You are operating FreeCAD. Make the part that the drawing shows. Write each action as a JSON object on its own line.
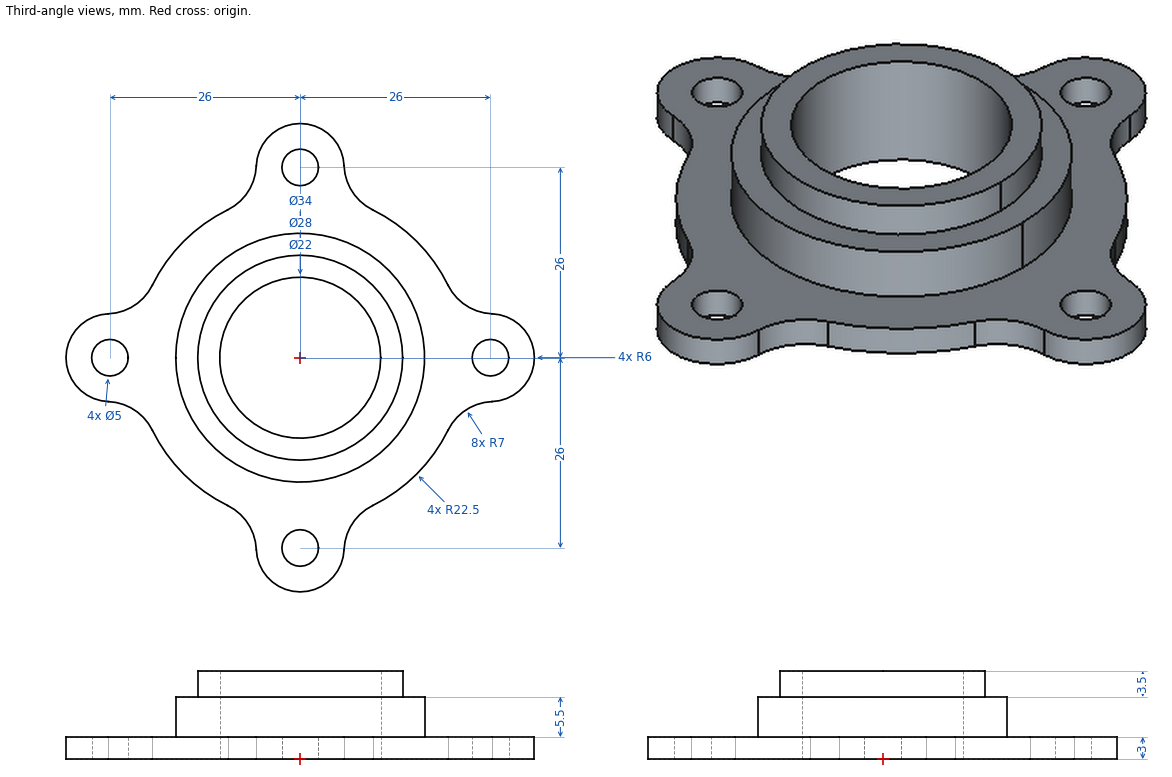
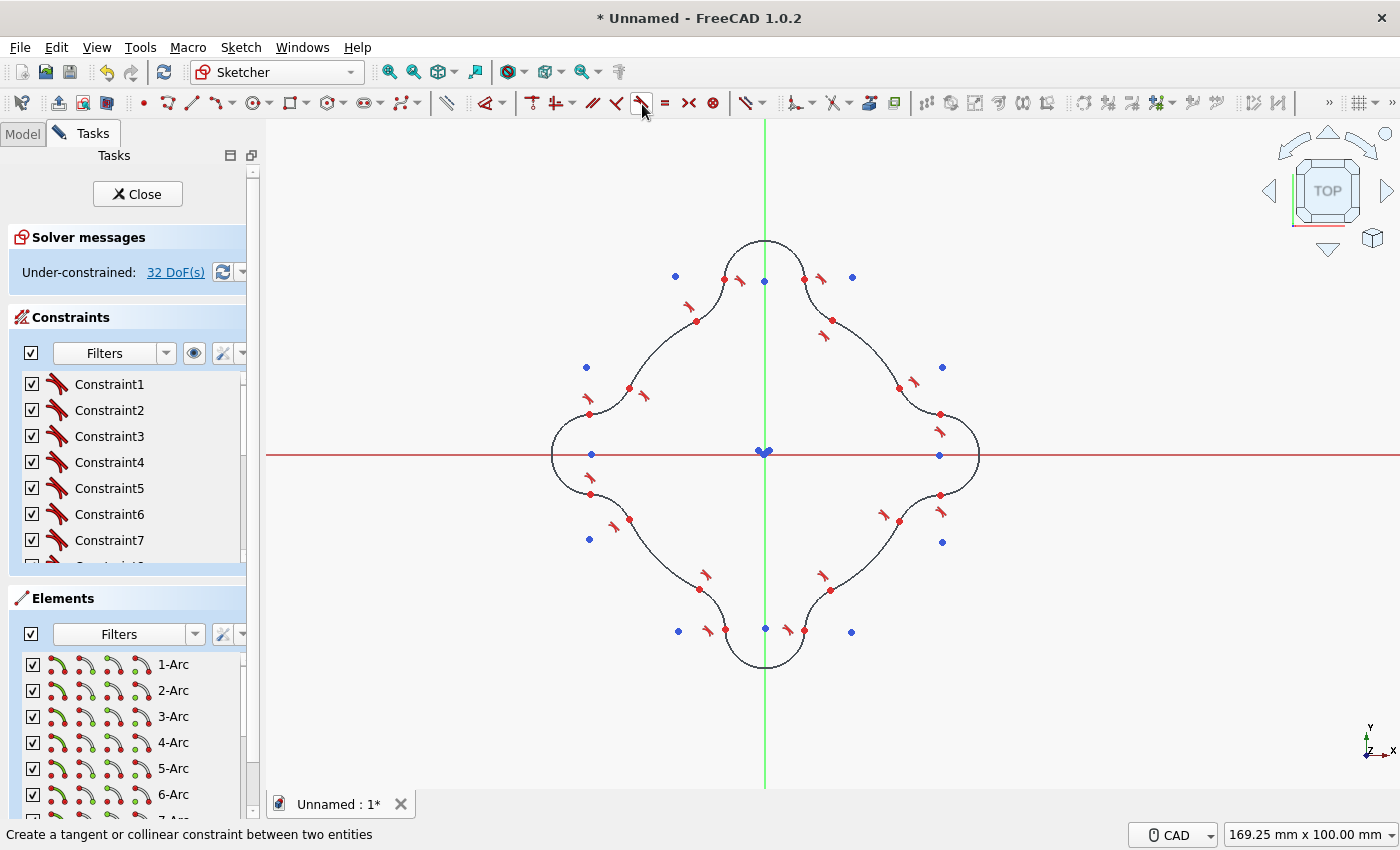
{"action": "left_click", "coordinate": [856, 575]}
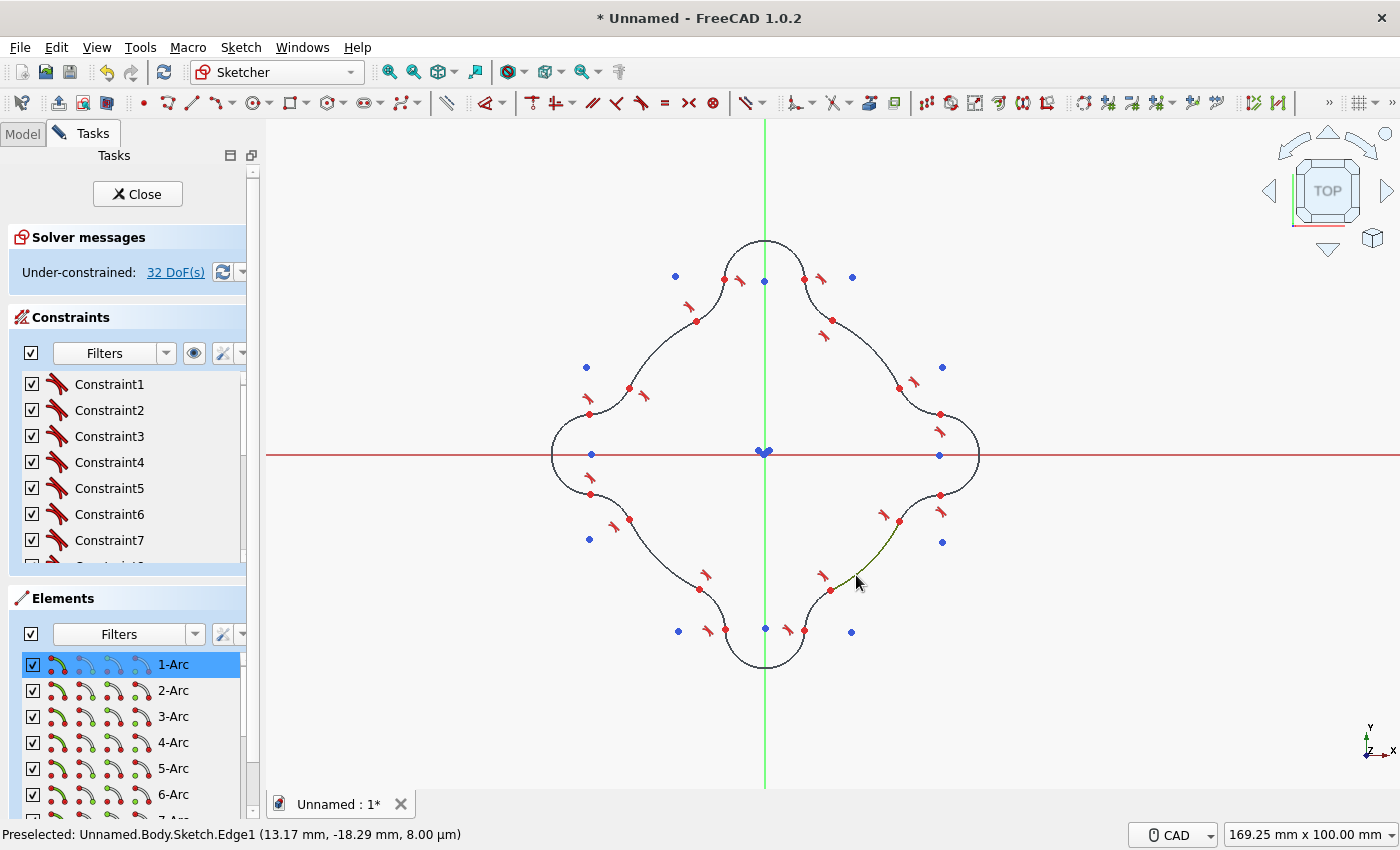
{"action": "left_click", "coordinate": [885, 363]}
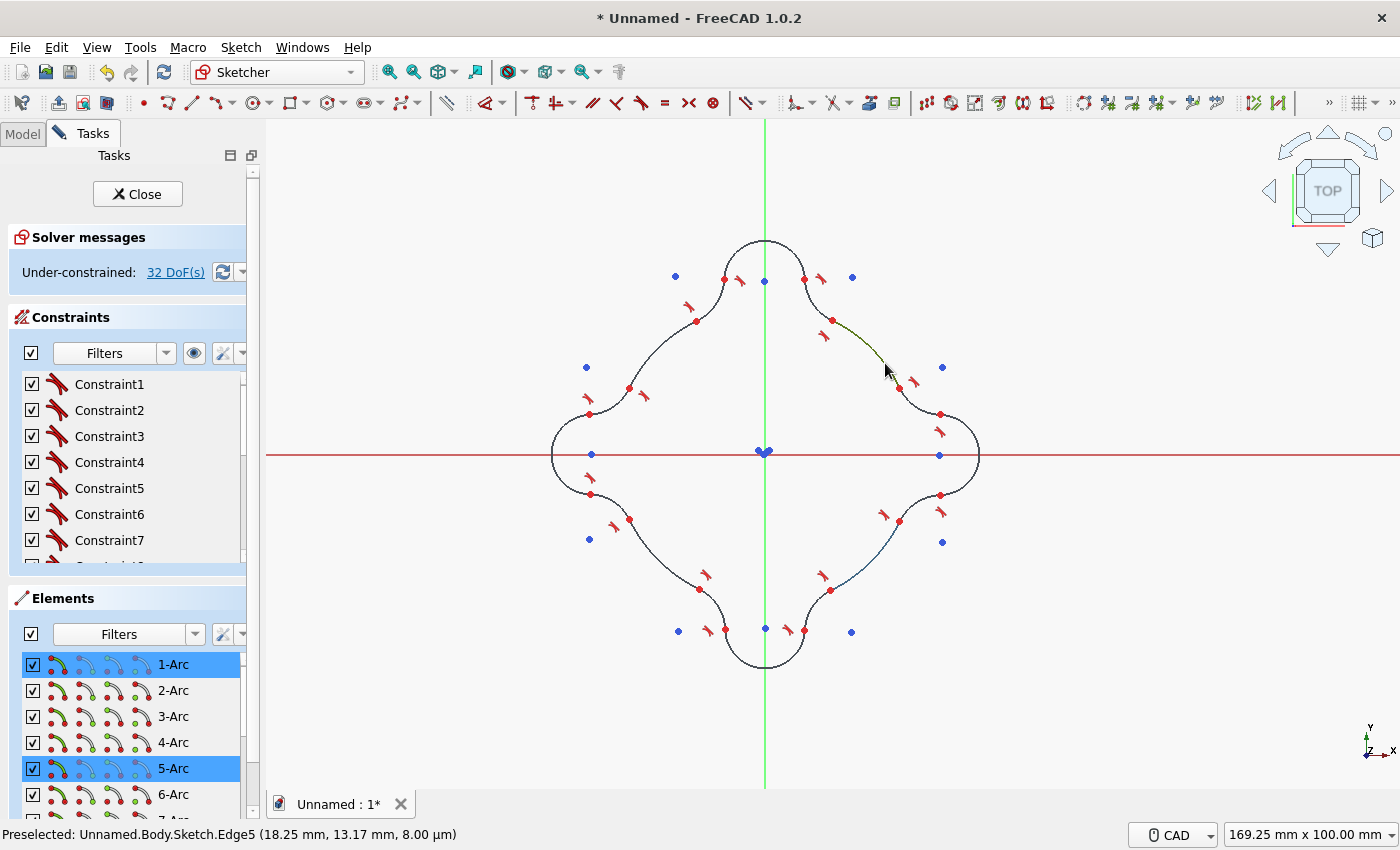
{"action": "left_click", "coordinate": [532, 104]}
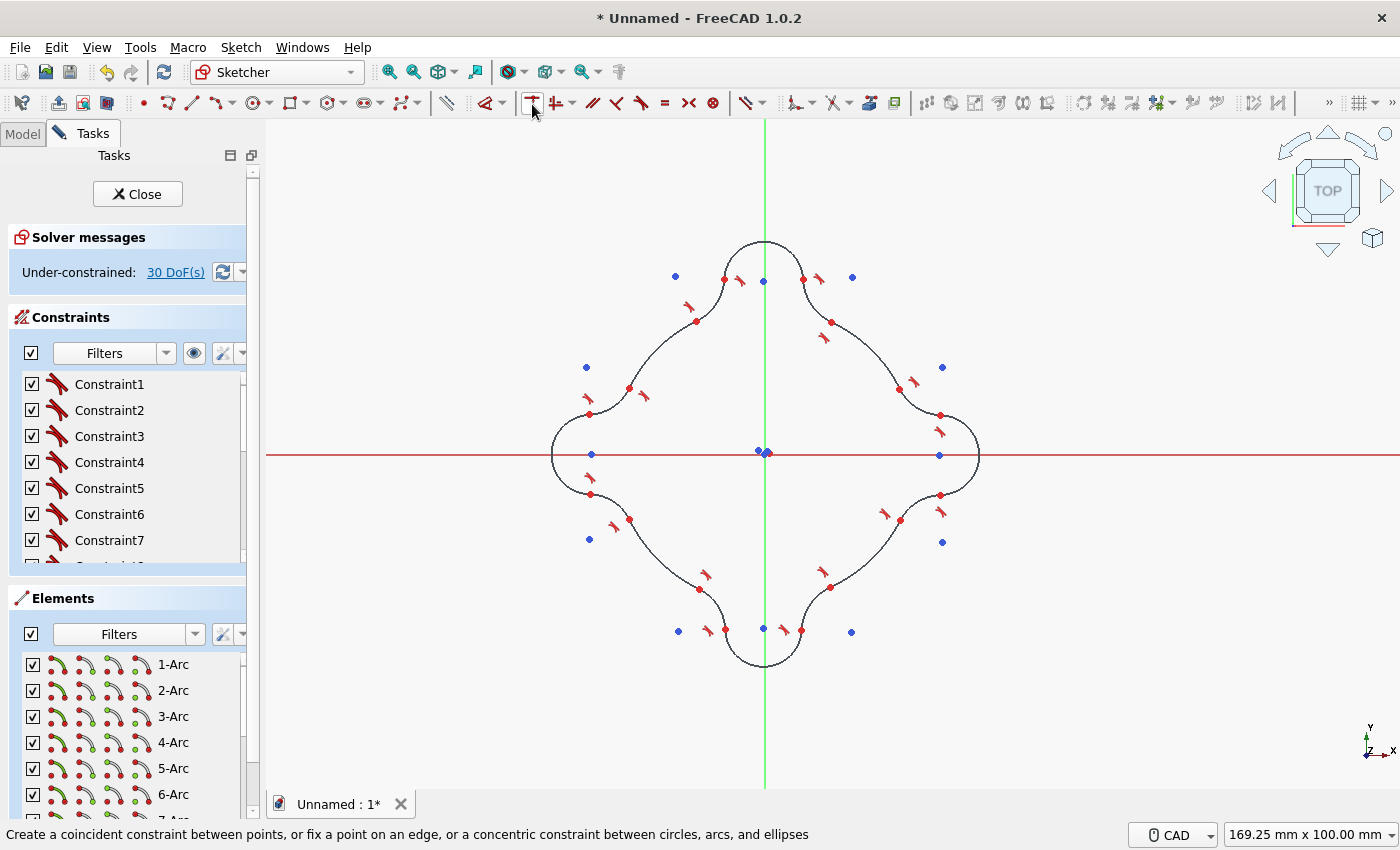
{"action": "left_click", "coordinate": [856, 572]}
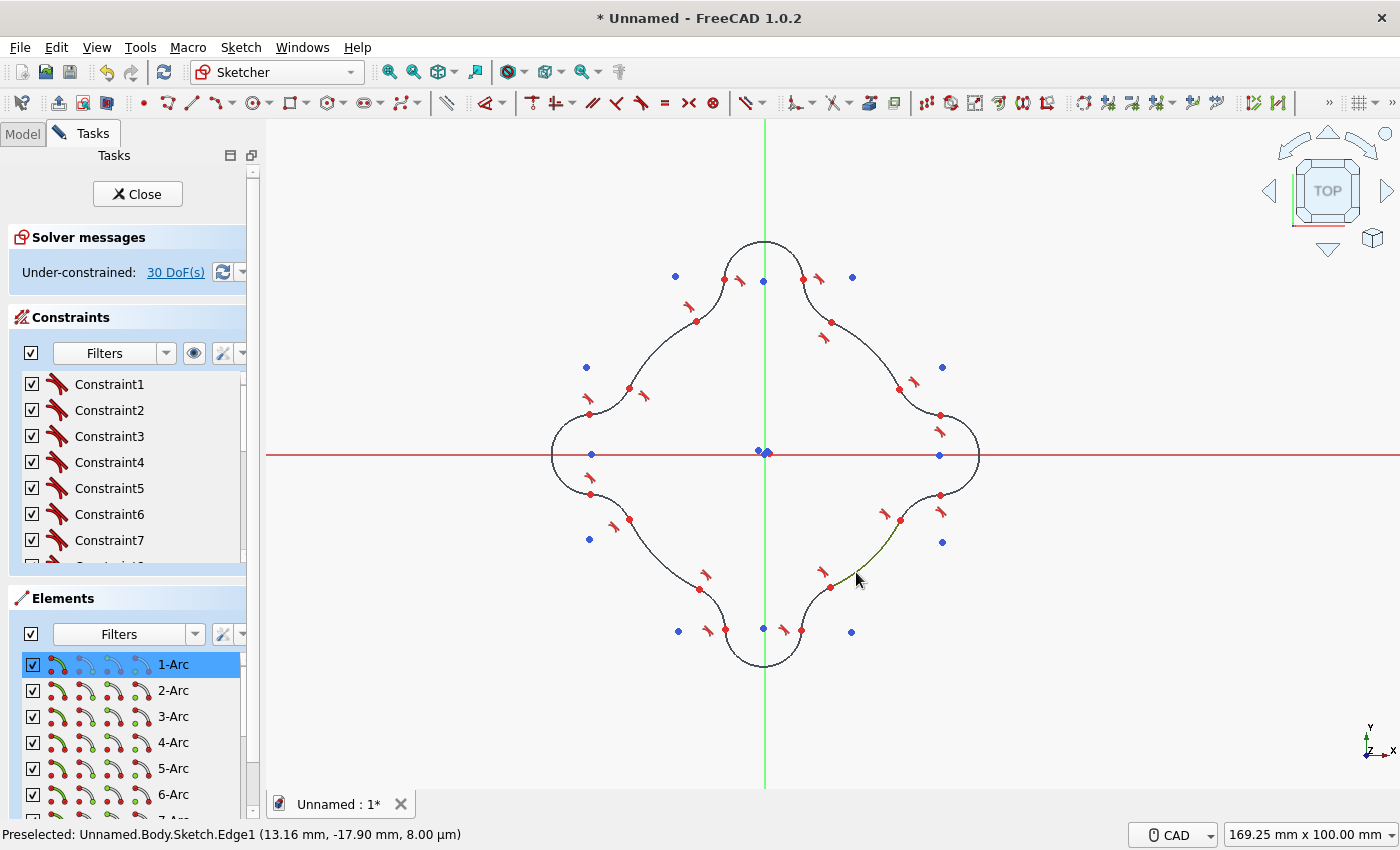
{"action": "left_click", "coordinate": [672, 336]}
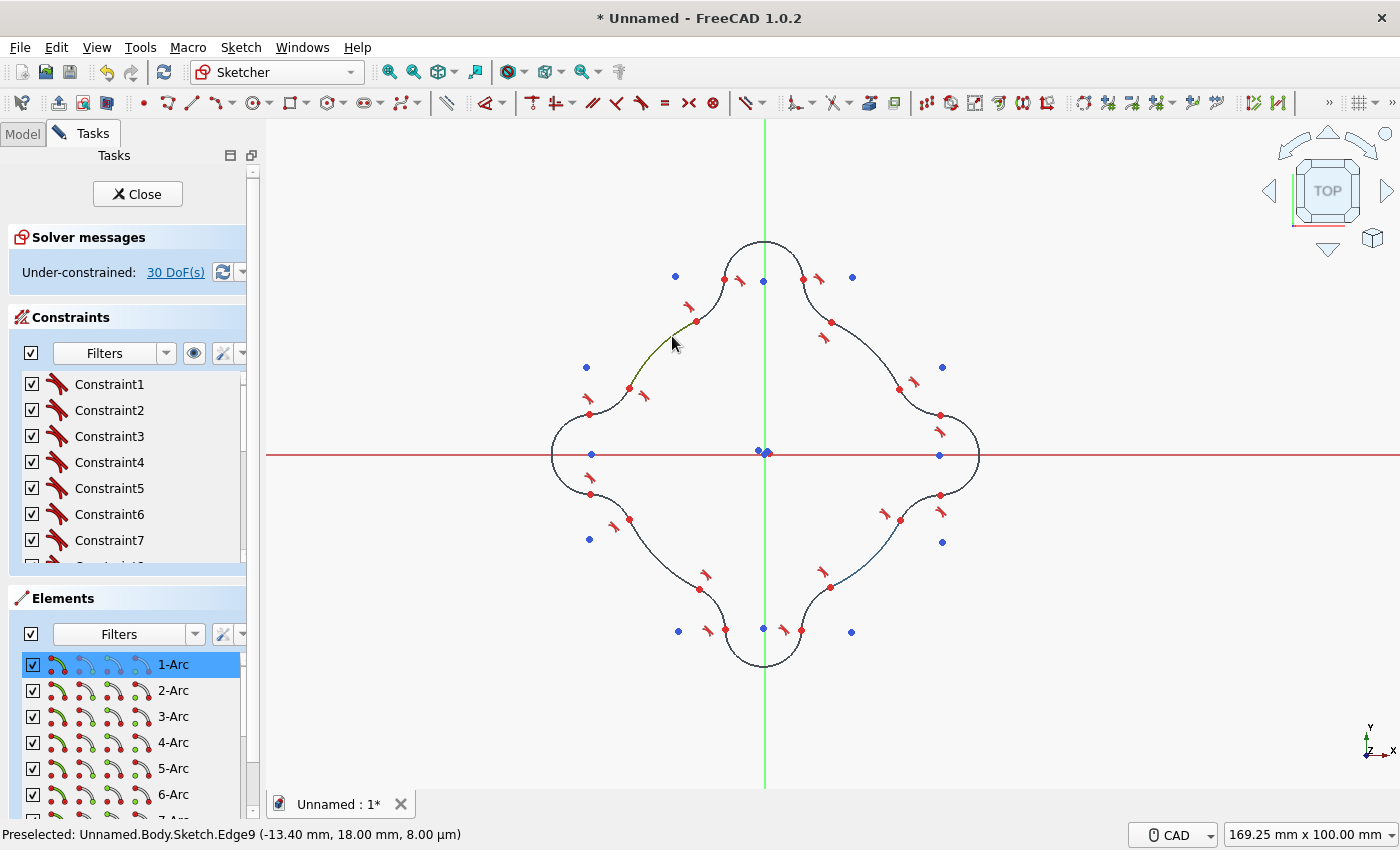
{"action": "left_click", "coordinate": [532, 104]}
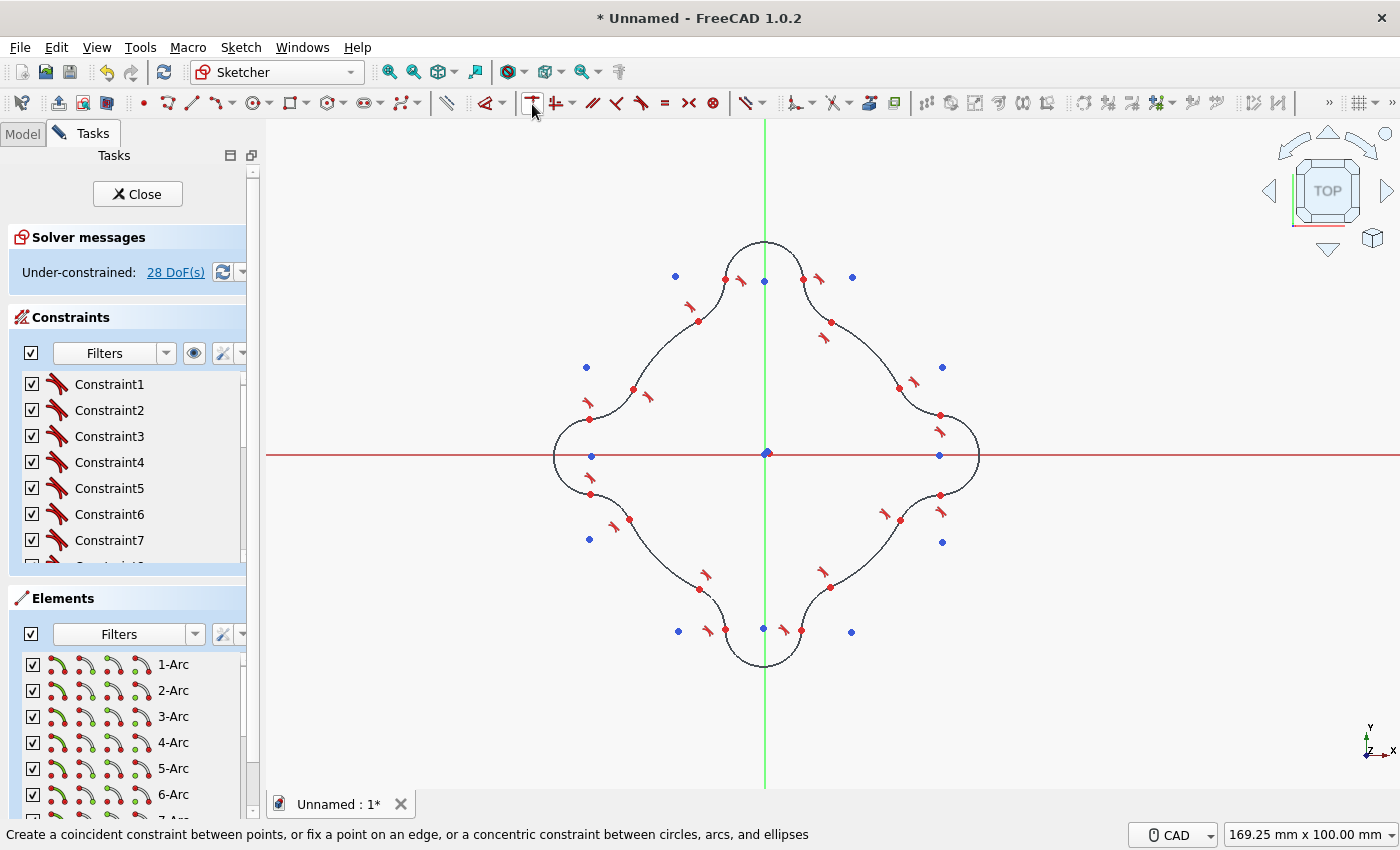
{"action": "left_click", "coordinate": [856, 572]}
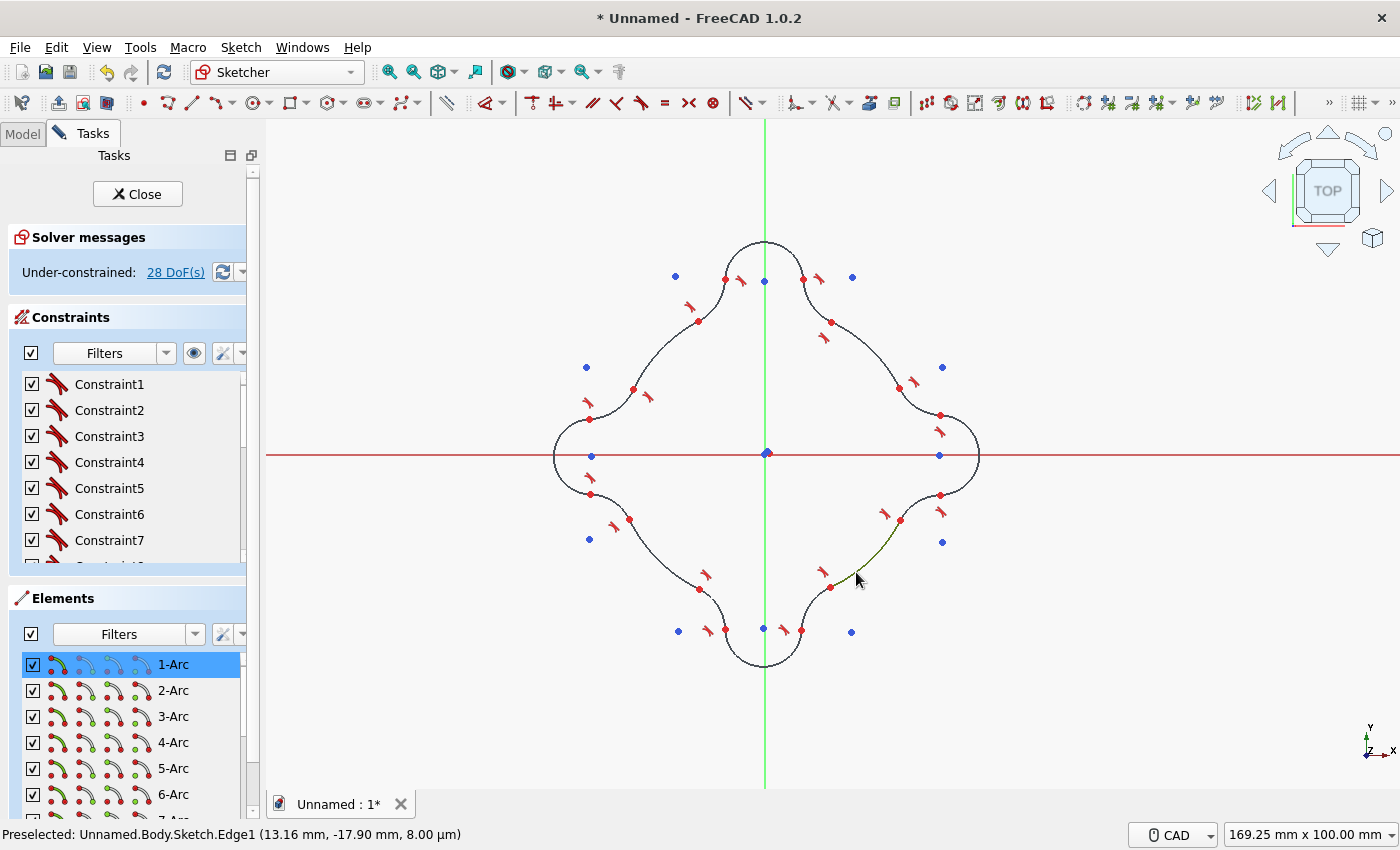
{"action": "left_click", "coordinate": [645, 545]}